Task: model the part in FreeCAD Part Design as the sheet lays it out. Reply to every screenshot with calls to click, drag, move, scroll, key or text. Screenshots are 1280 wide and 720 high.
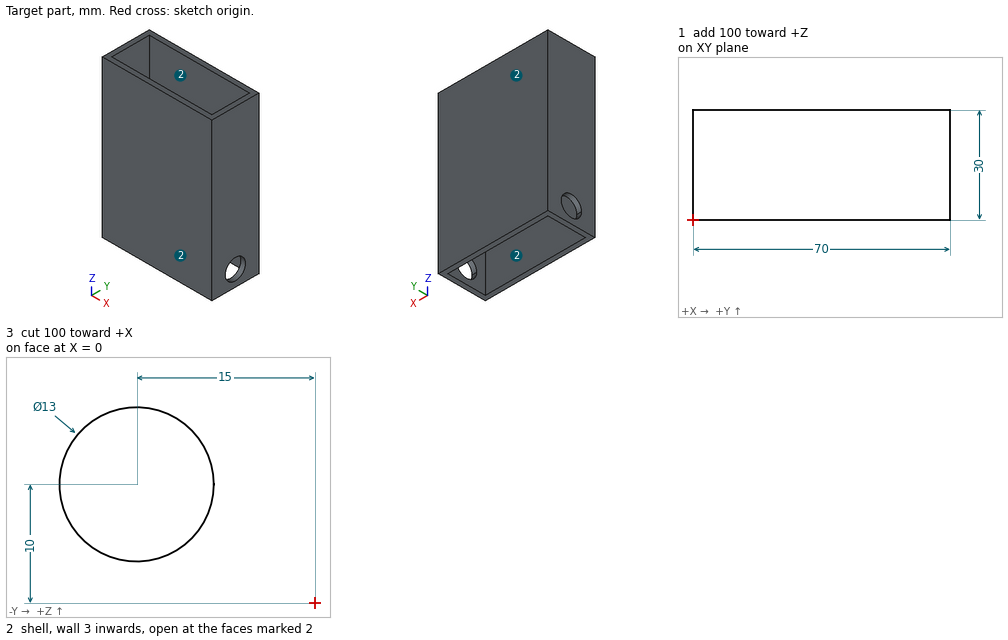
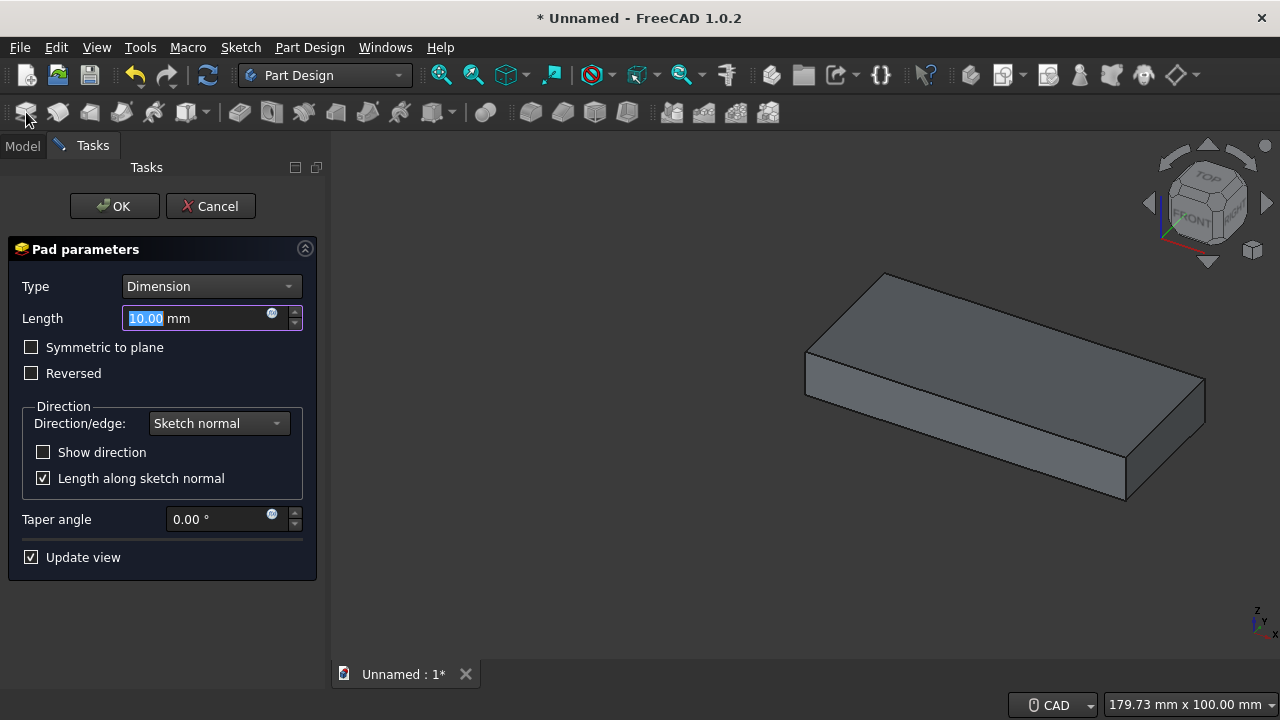
text(100)
key(Tab)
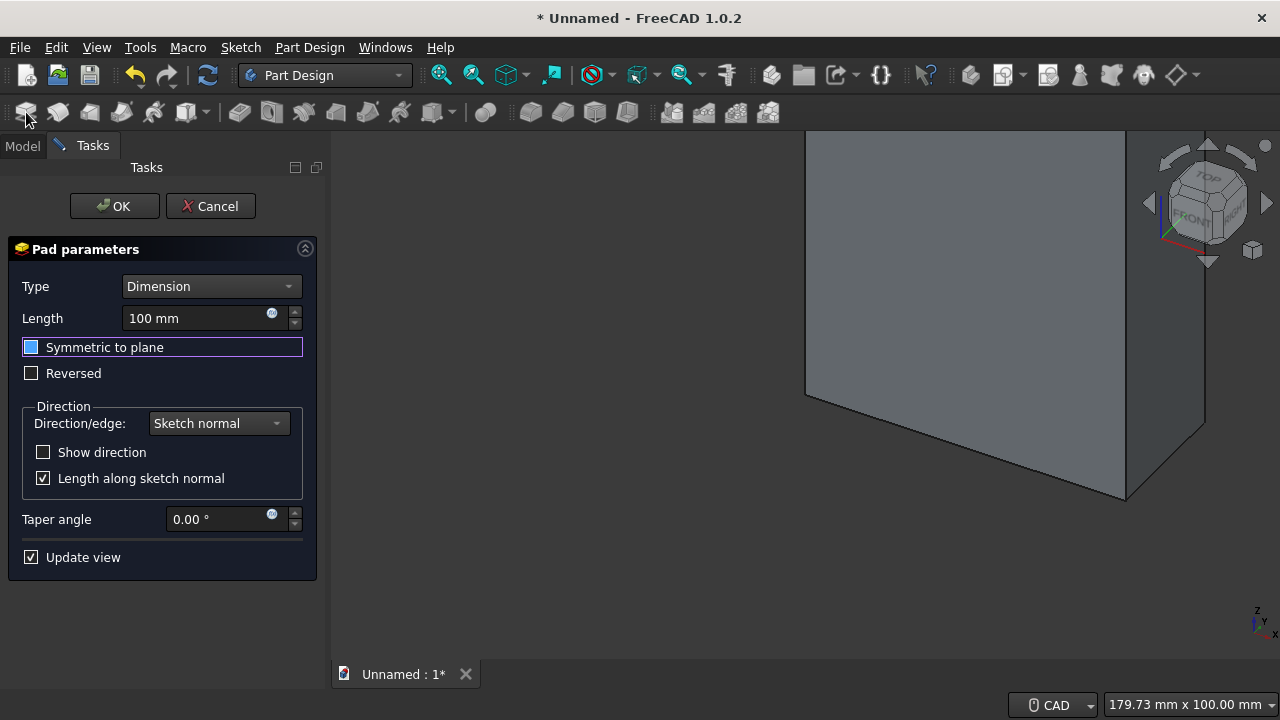
click(115, 206)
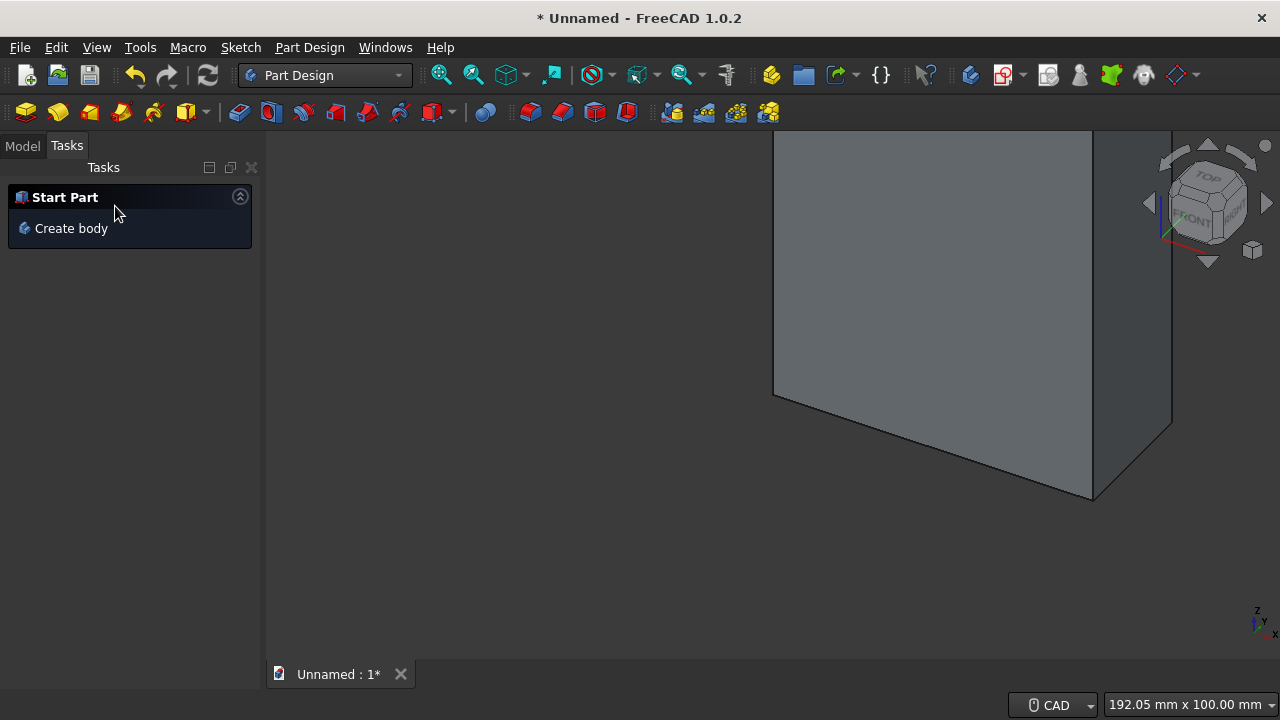
click(442, 76)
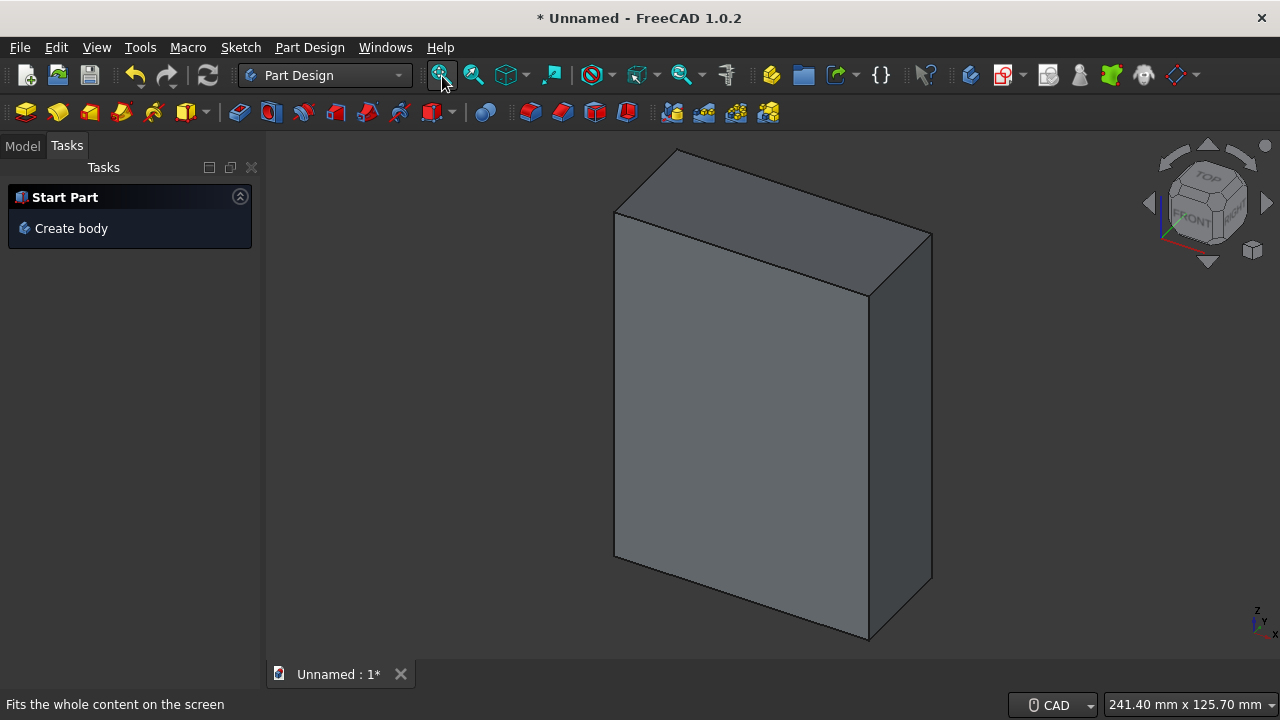
click(846, 246)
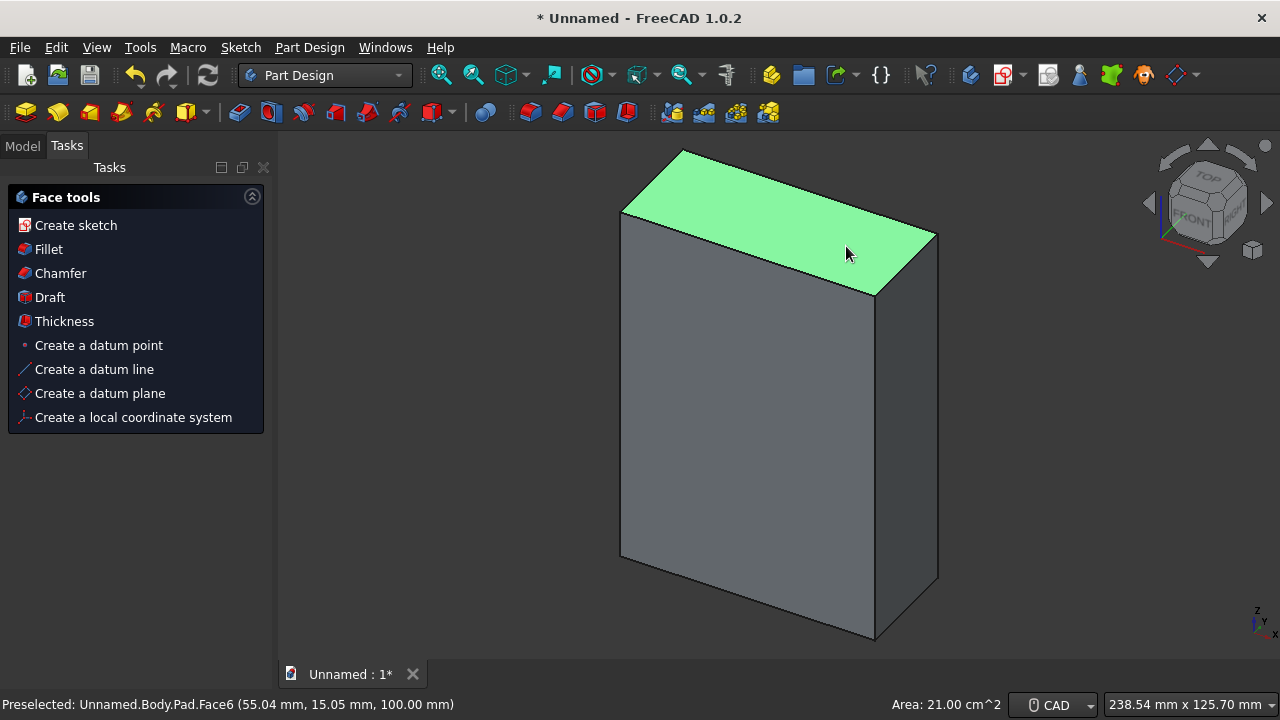
key(0)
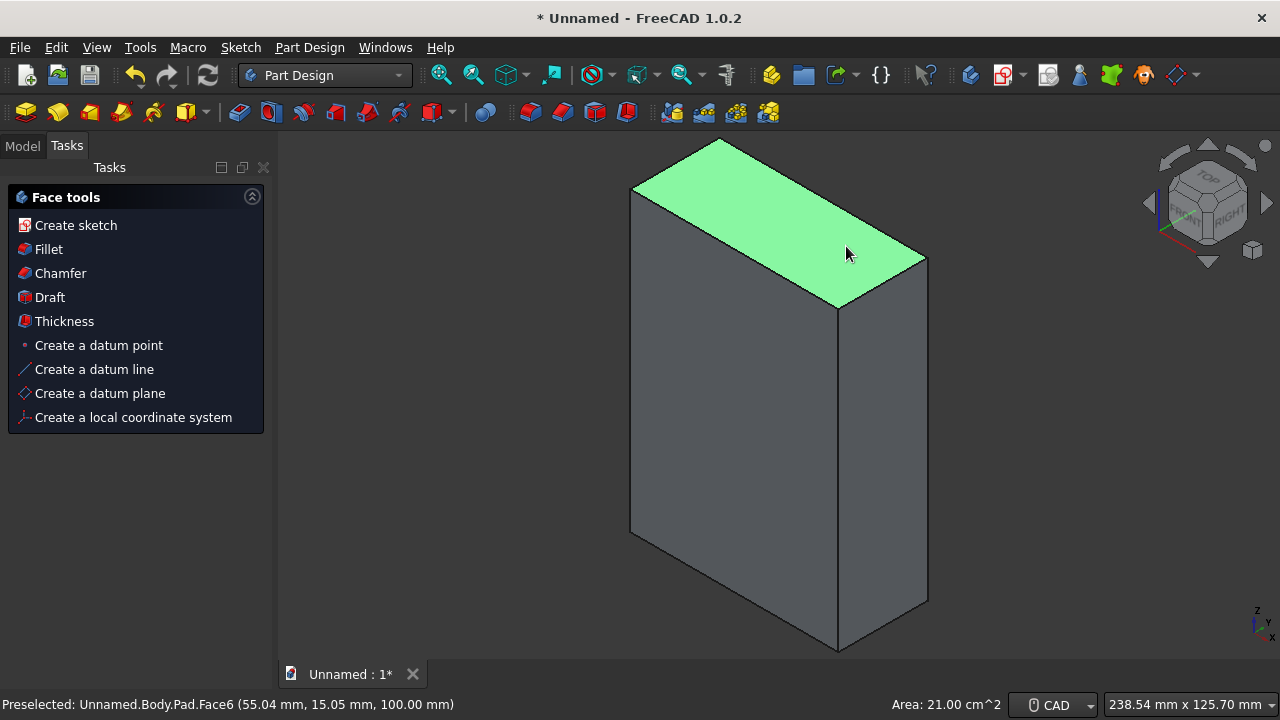
key(2)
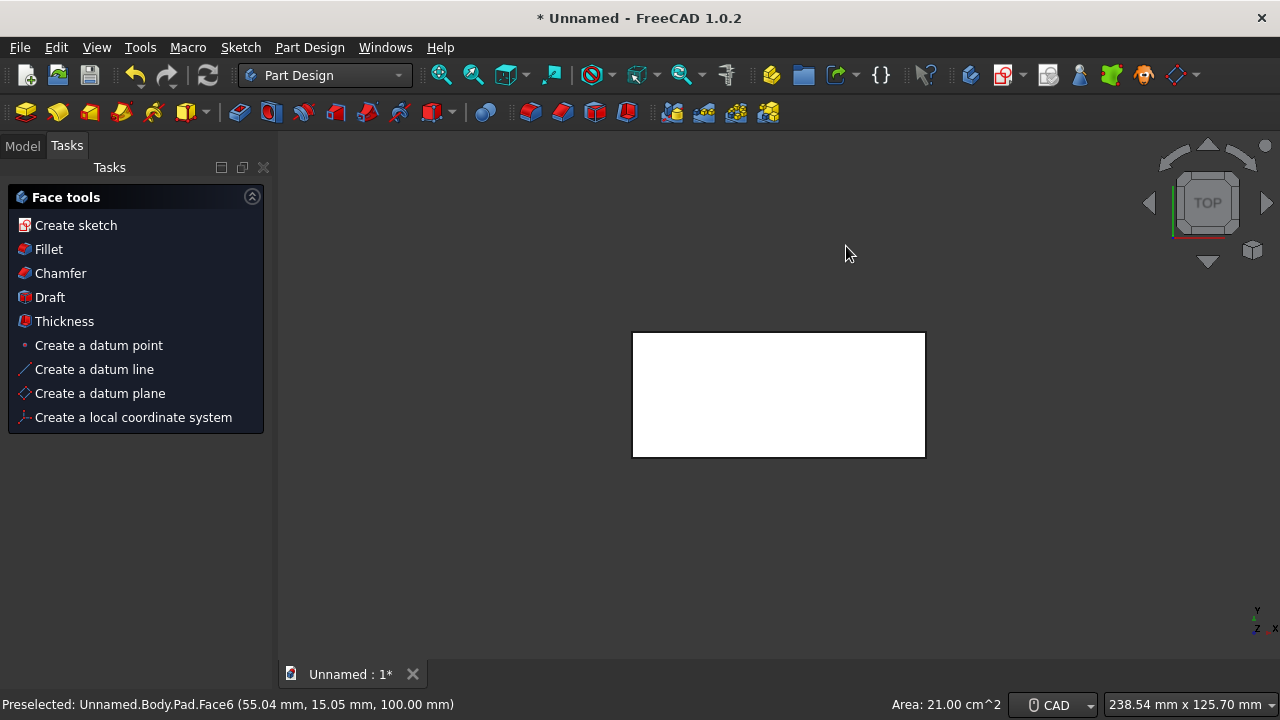
click(442, 76)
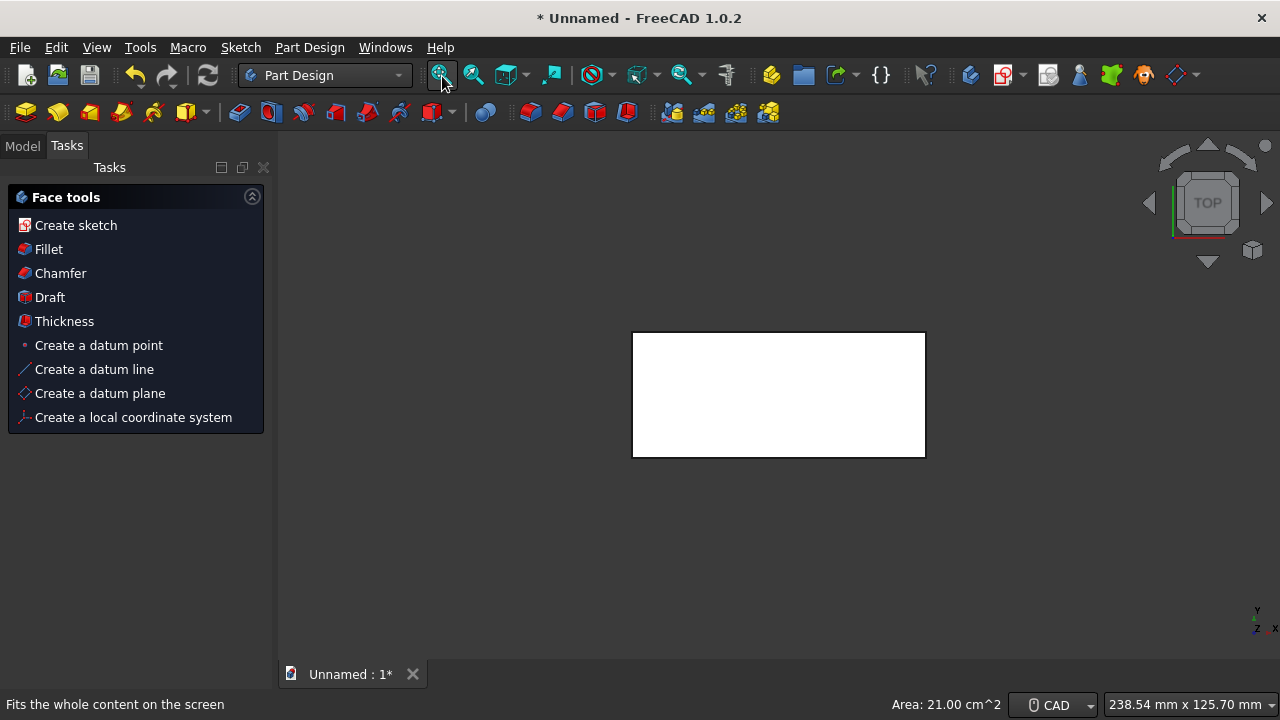
key(1)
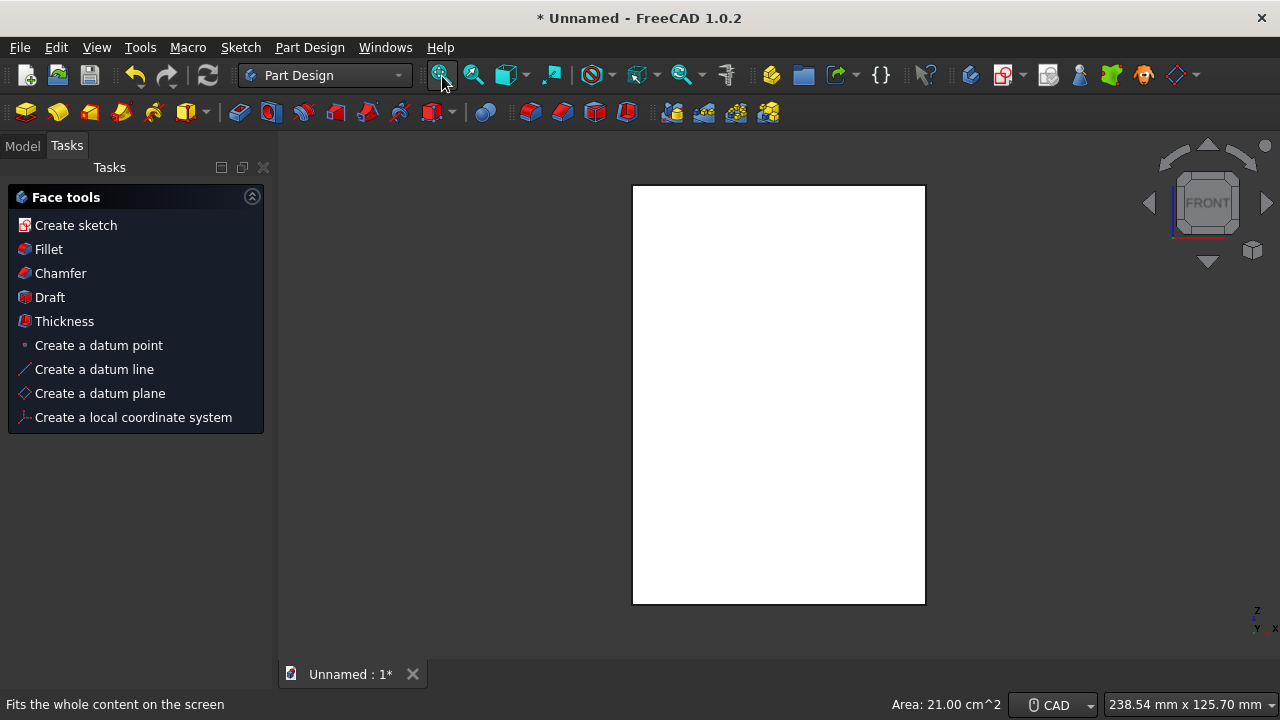
key(3)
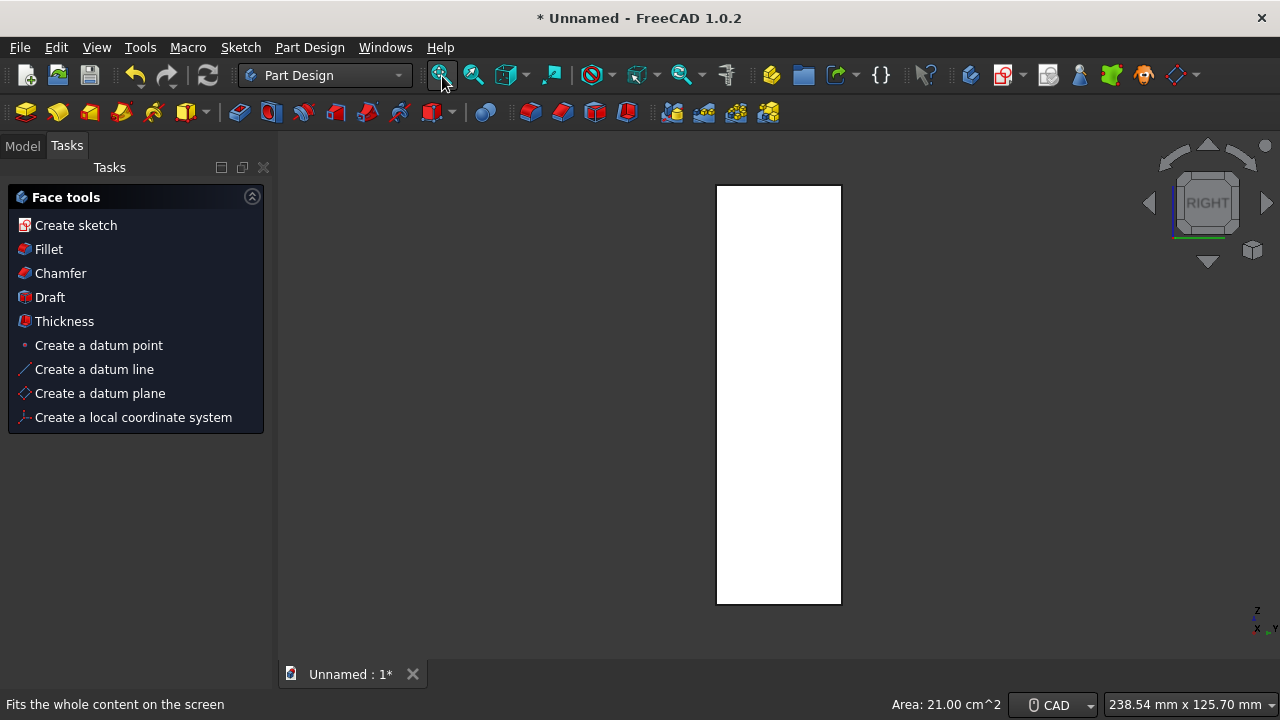
key(5)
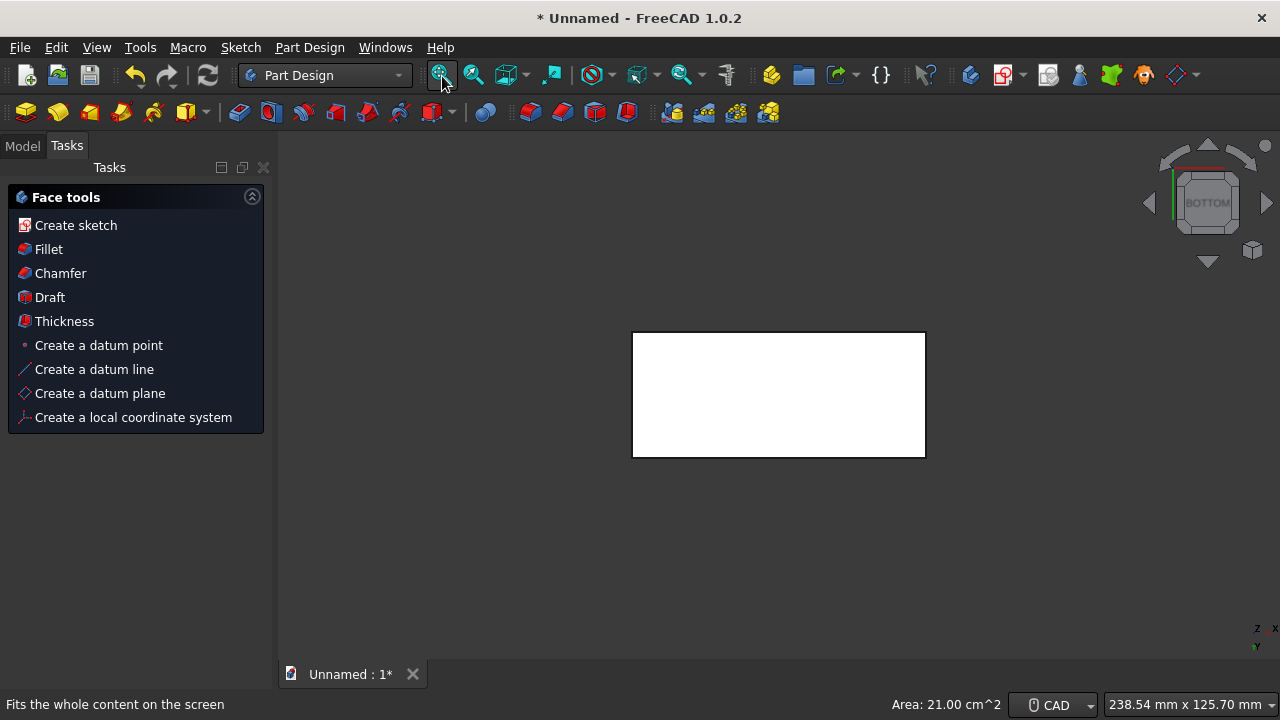
click(442, 76)